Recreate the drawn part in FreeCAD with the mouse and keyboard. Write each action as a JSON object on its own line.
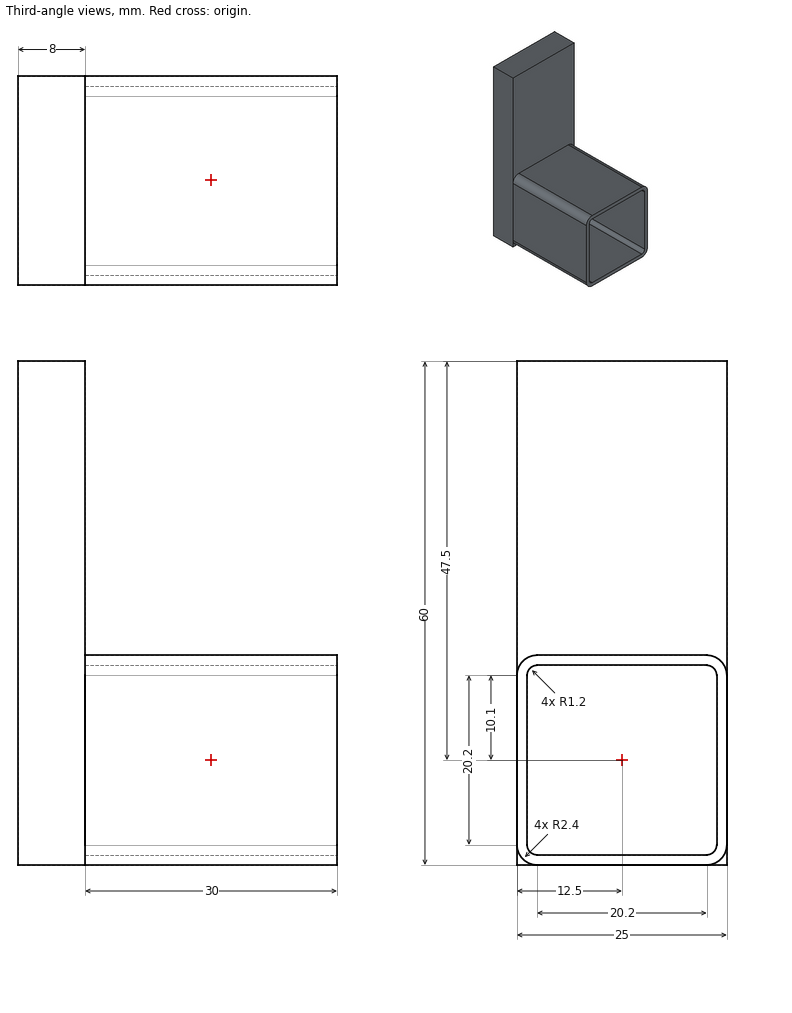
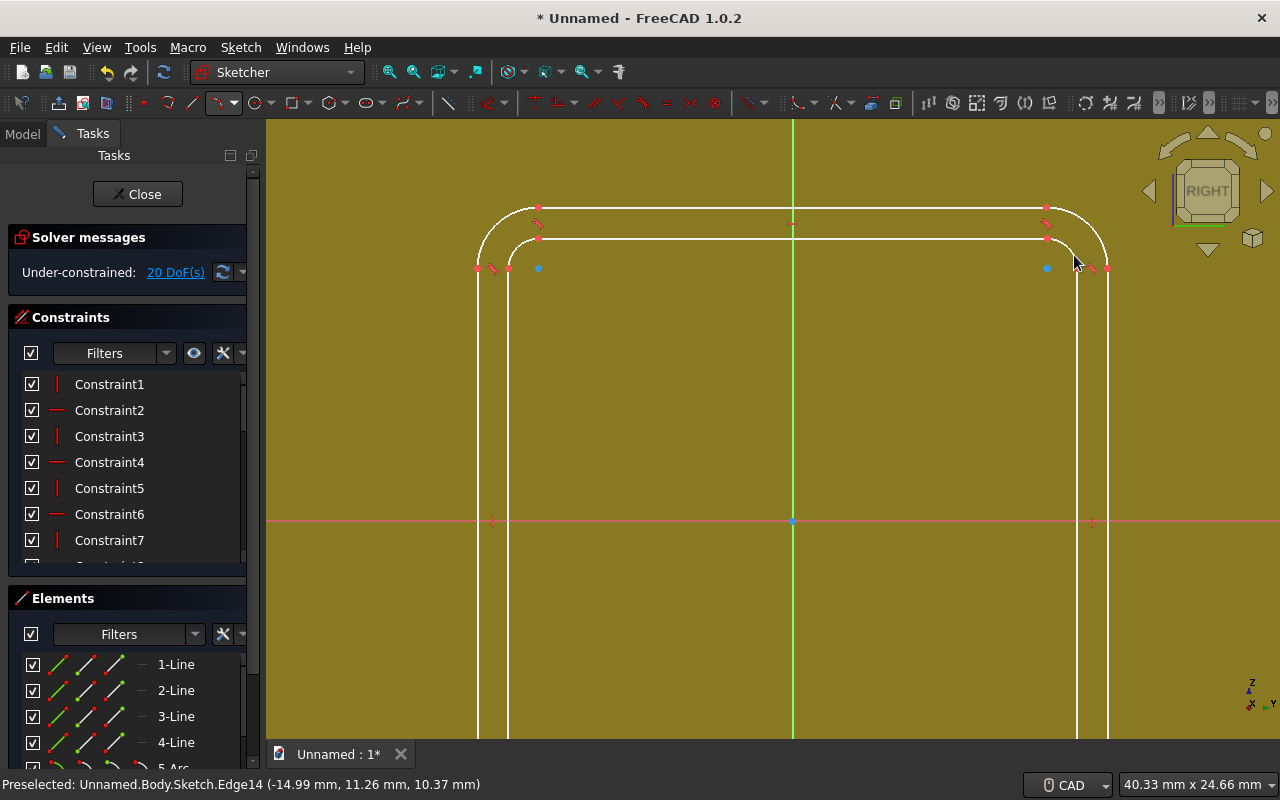
{"action": "left_click", "coordinate": [1077, 421]}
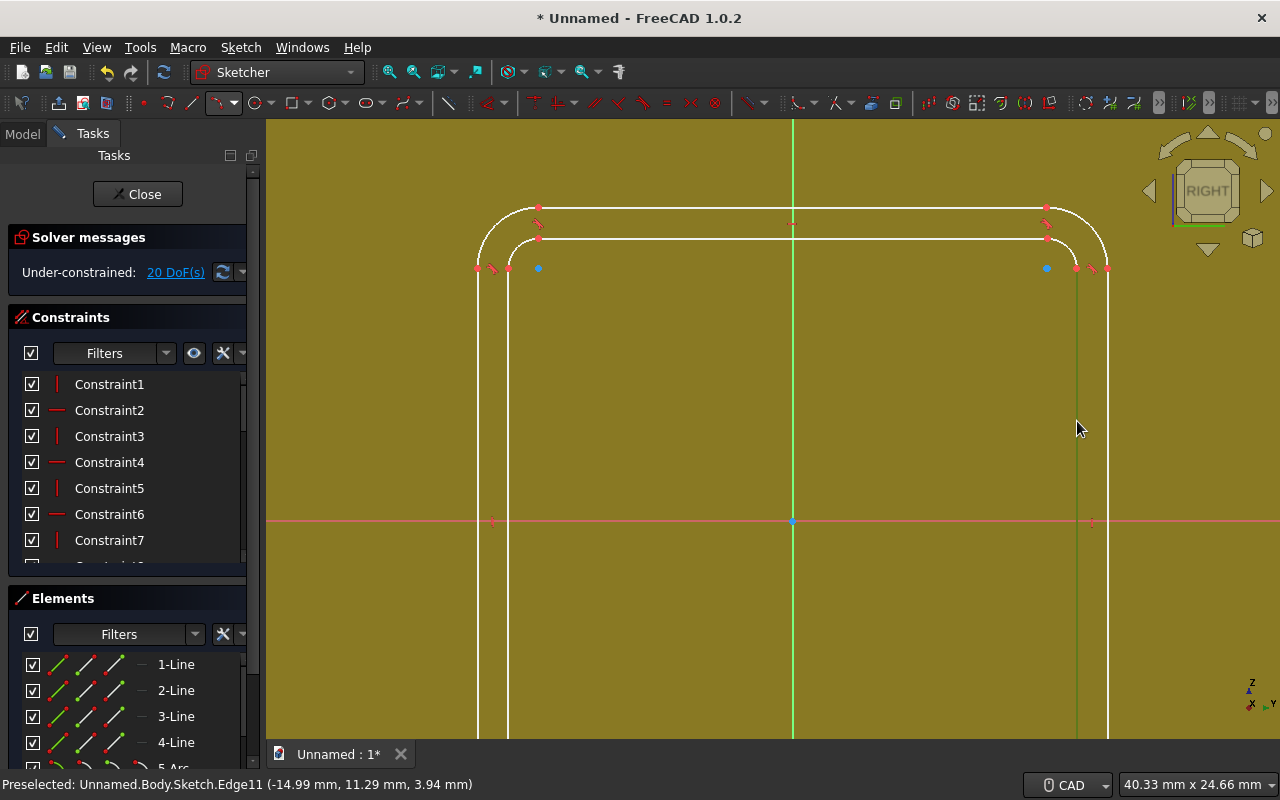
{"action": "left_click", "coordinate": [1074, 255]}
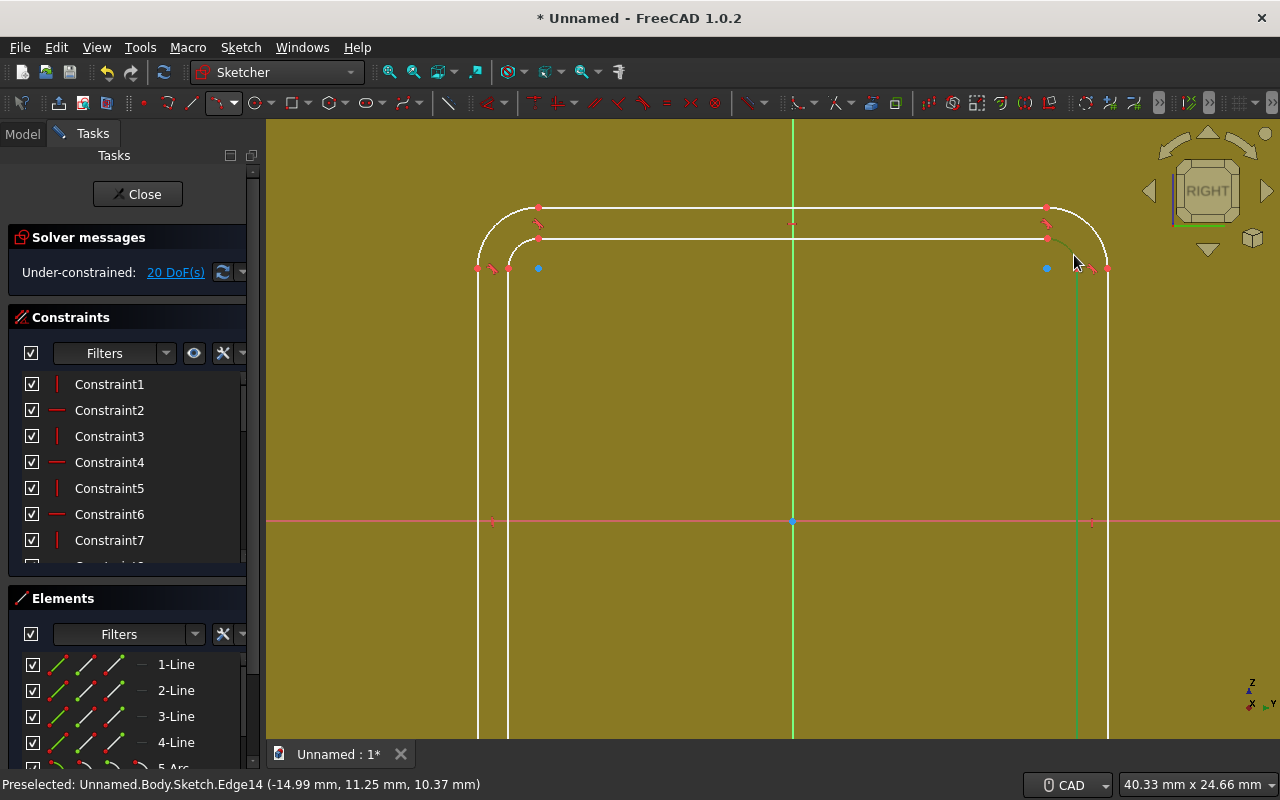
{"action": "key", "text": "t"}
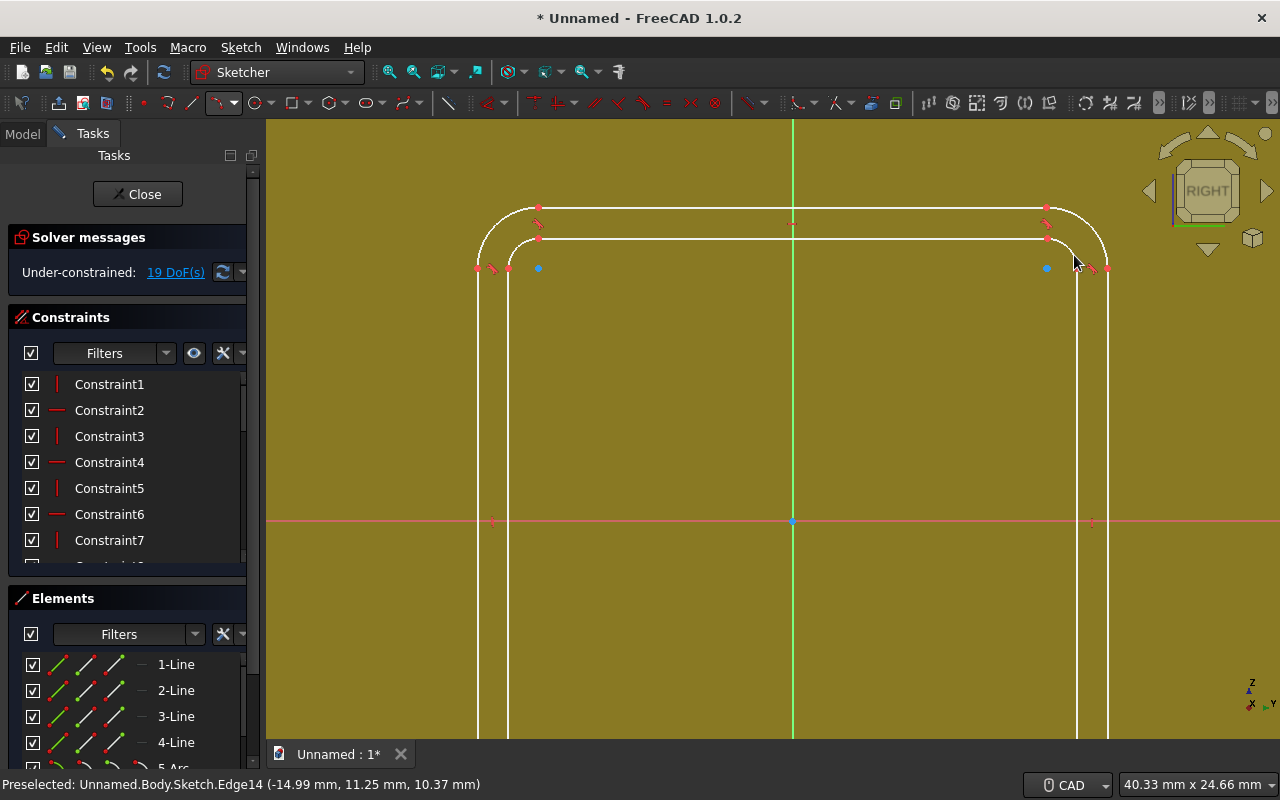
{"action": "left_click", "coordinate": [1077, 421]}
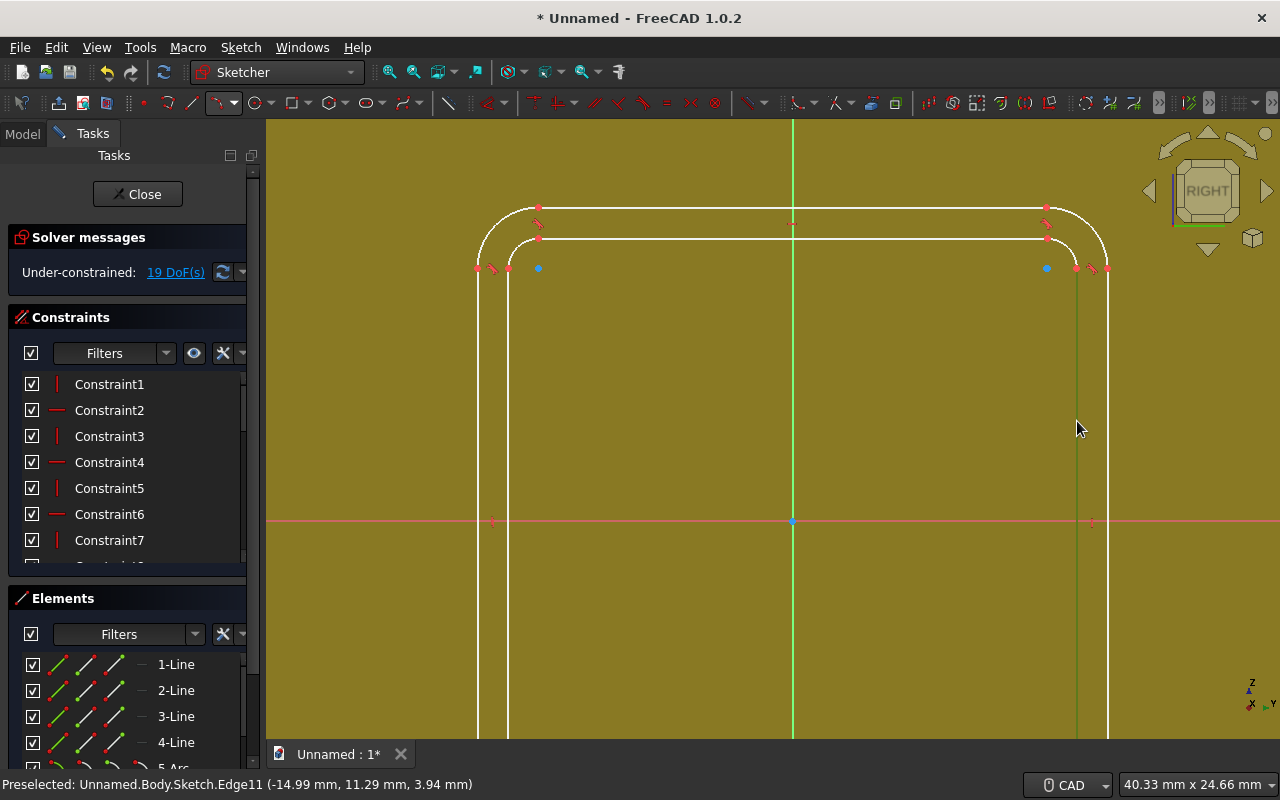
{"action": "scroll", "coordinate": [525, 242], "scroll_direction": "down", "scroll_amount": 2}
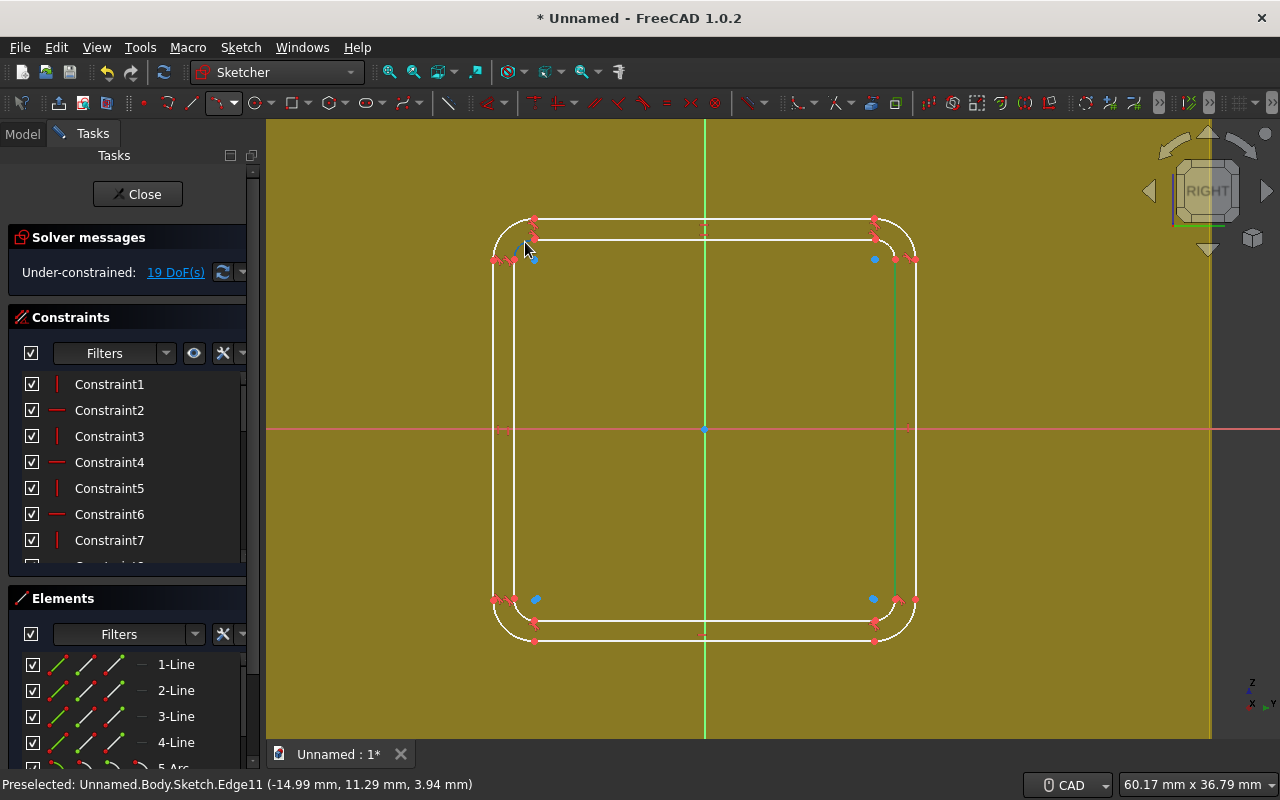
{"action": "scroll", "coordinate": [884, 618], "scroll_direction": "up", "scroll_amount": 2}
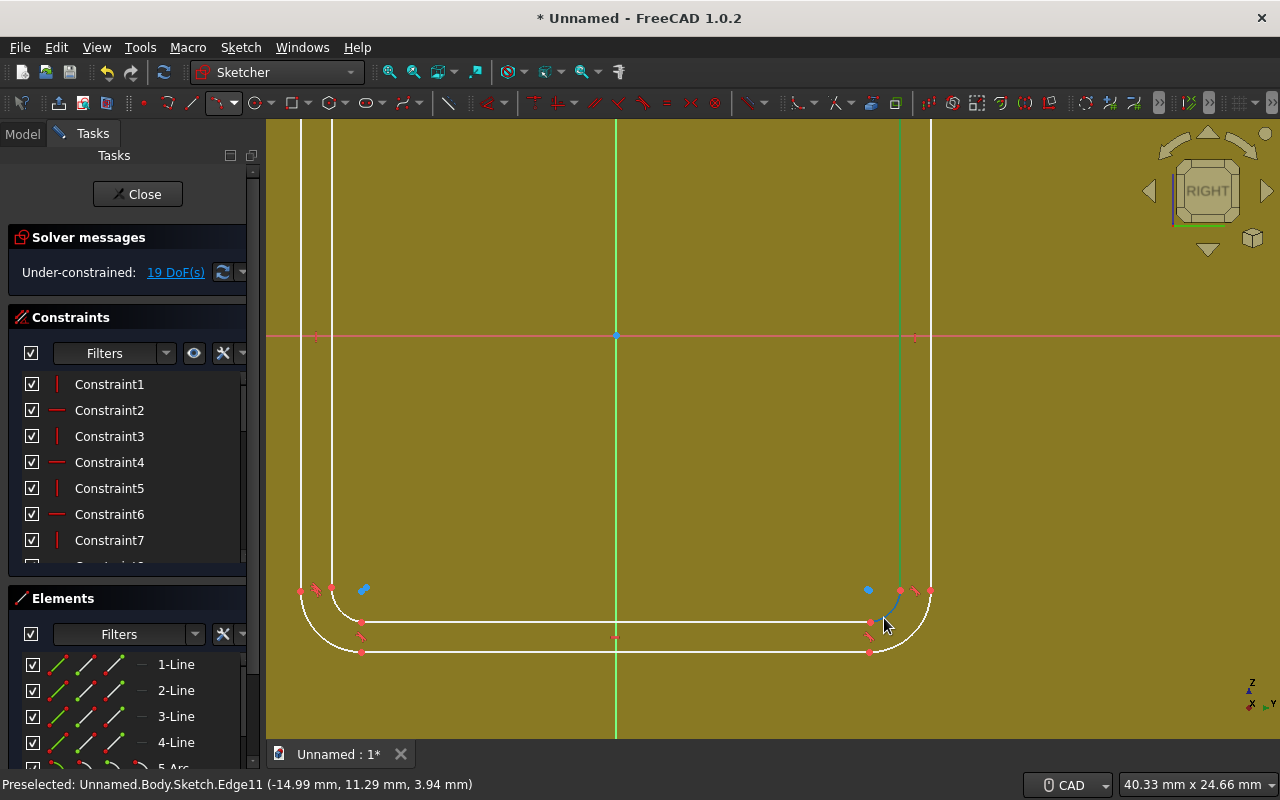
{"action": "left_click", "coordinate": [884, 618]}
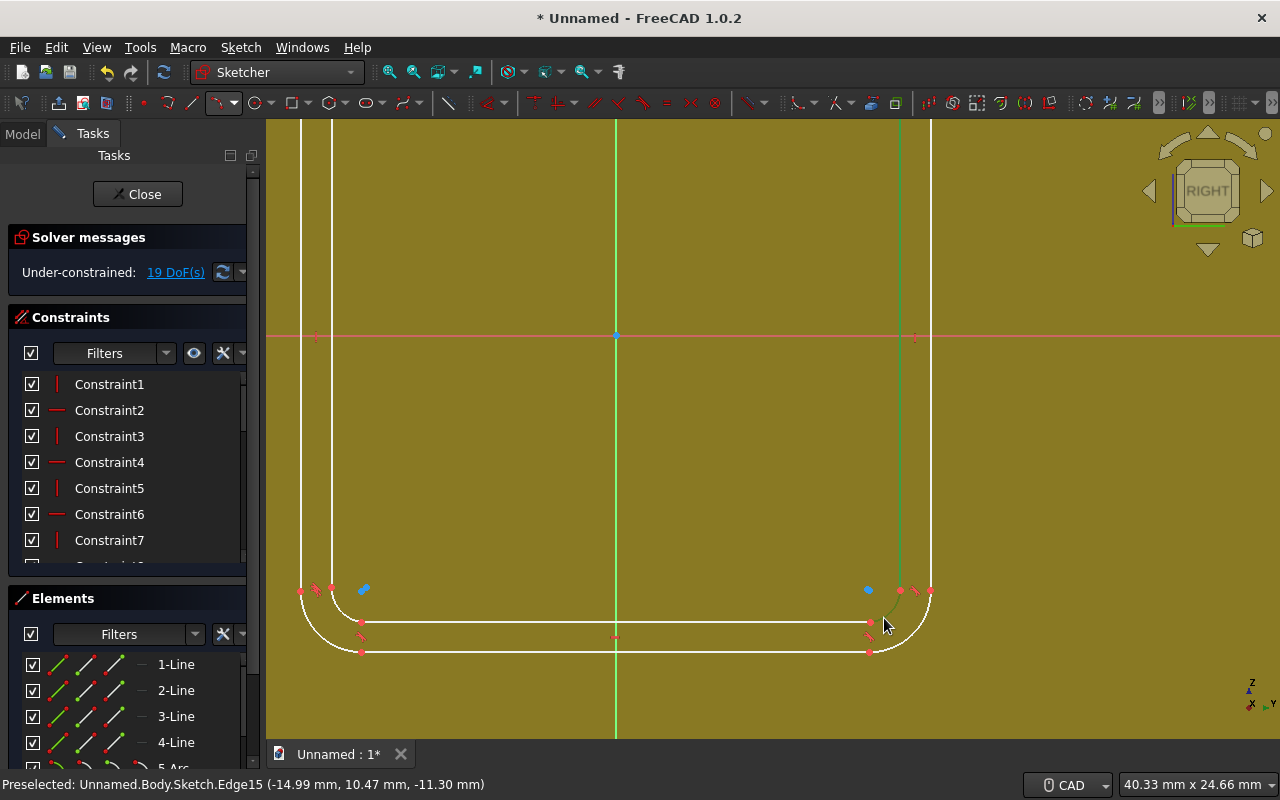
{"action": "key", "text": "t"}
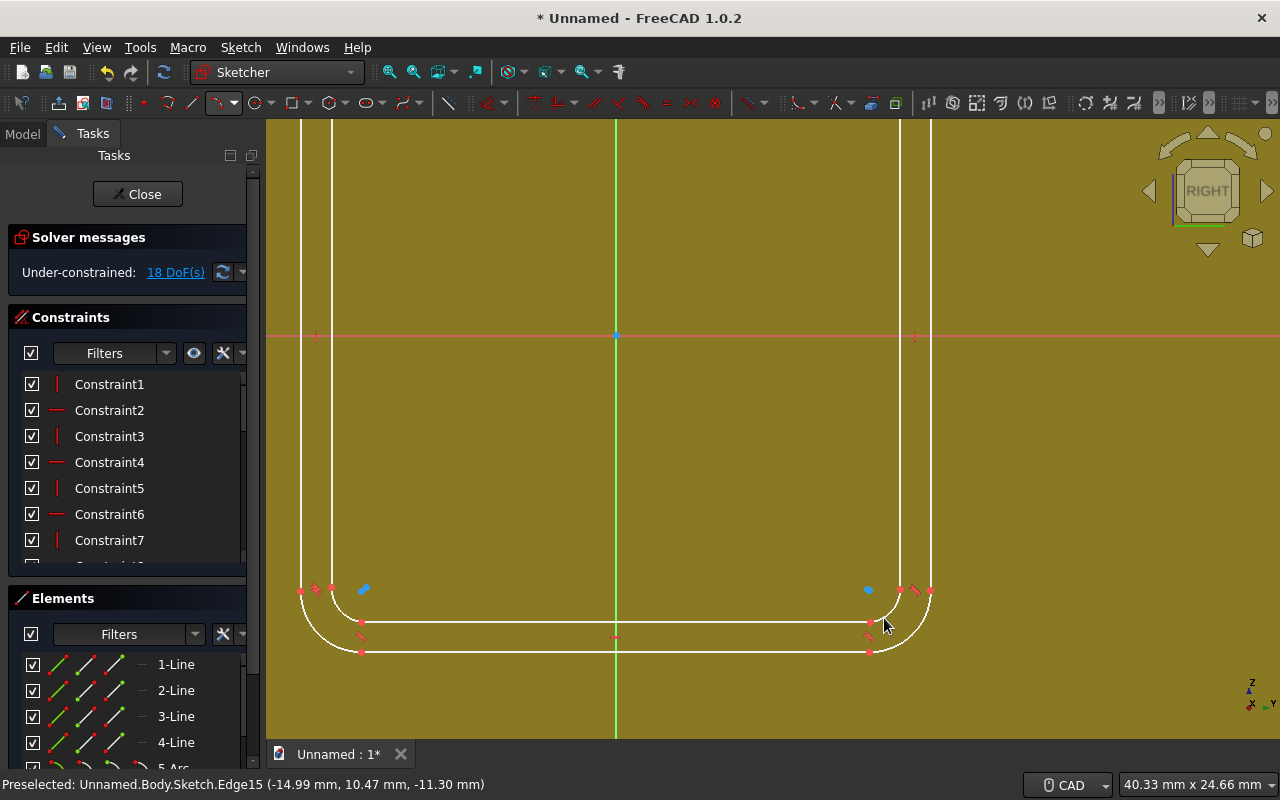
{"action": "left_click", "coordinate": [718, 622]}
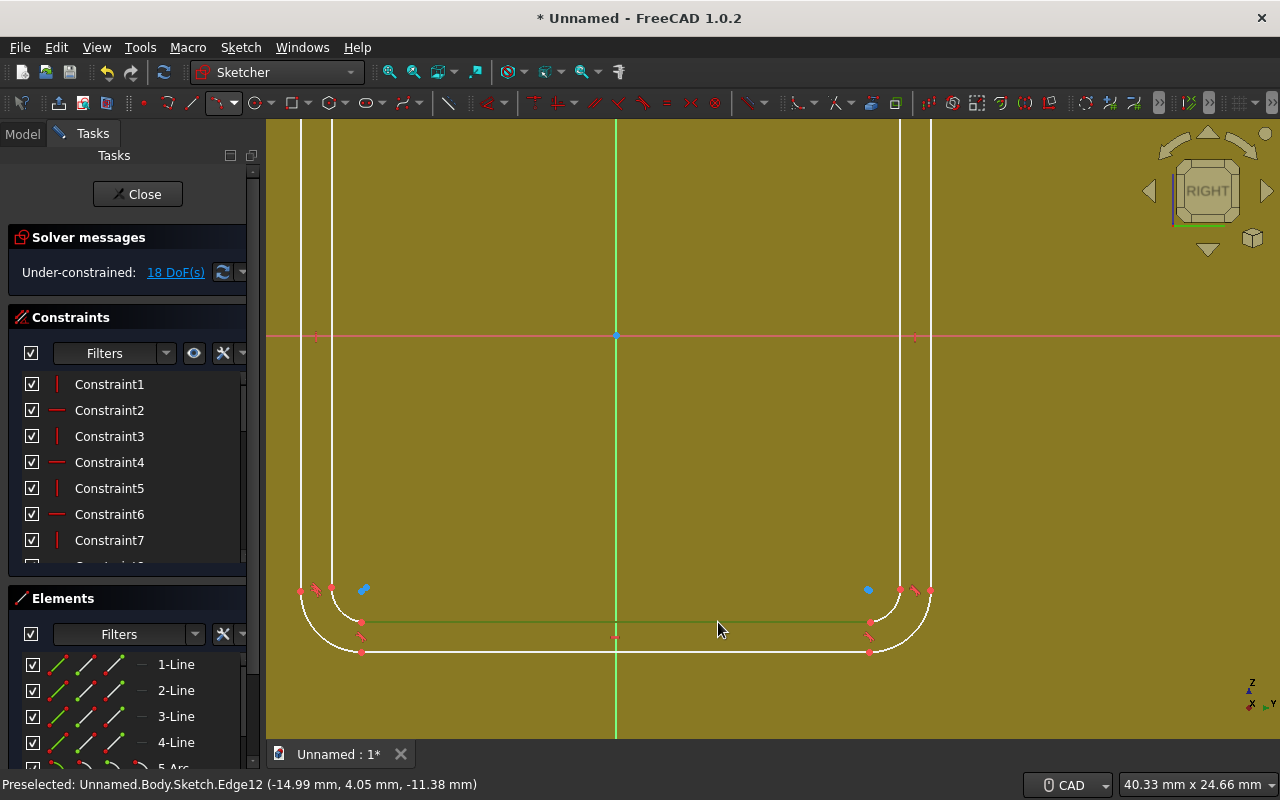
{"action": "left_click", "coordinate": [884, 618]}